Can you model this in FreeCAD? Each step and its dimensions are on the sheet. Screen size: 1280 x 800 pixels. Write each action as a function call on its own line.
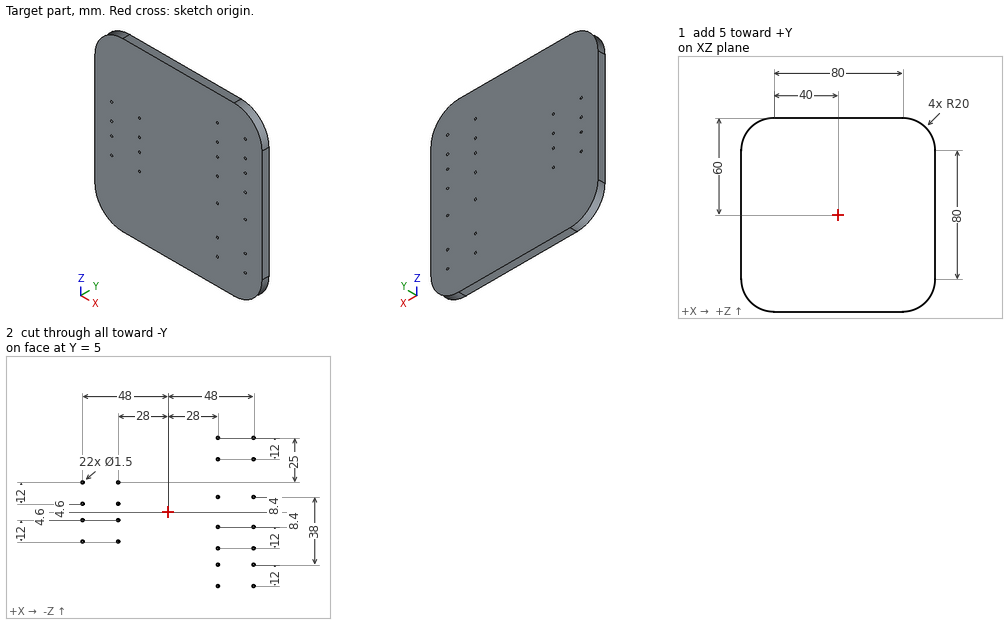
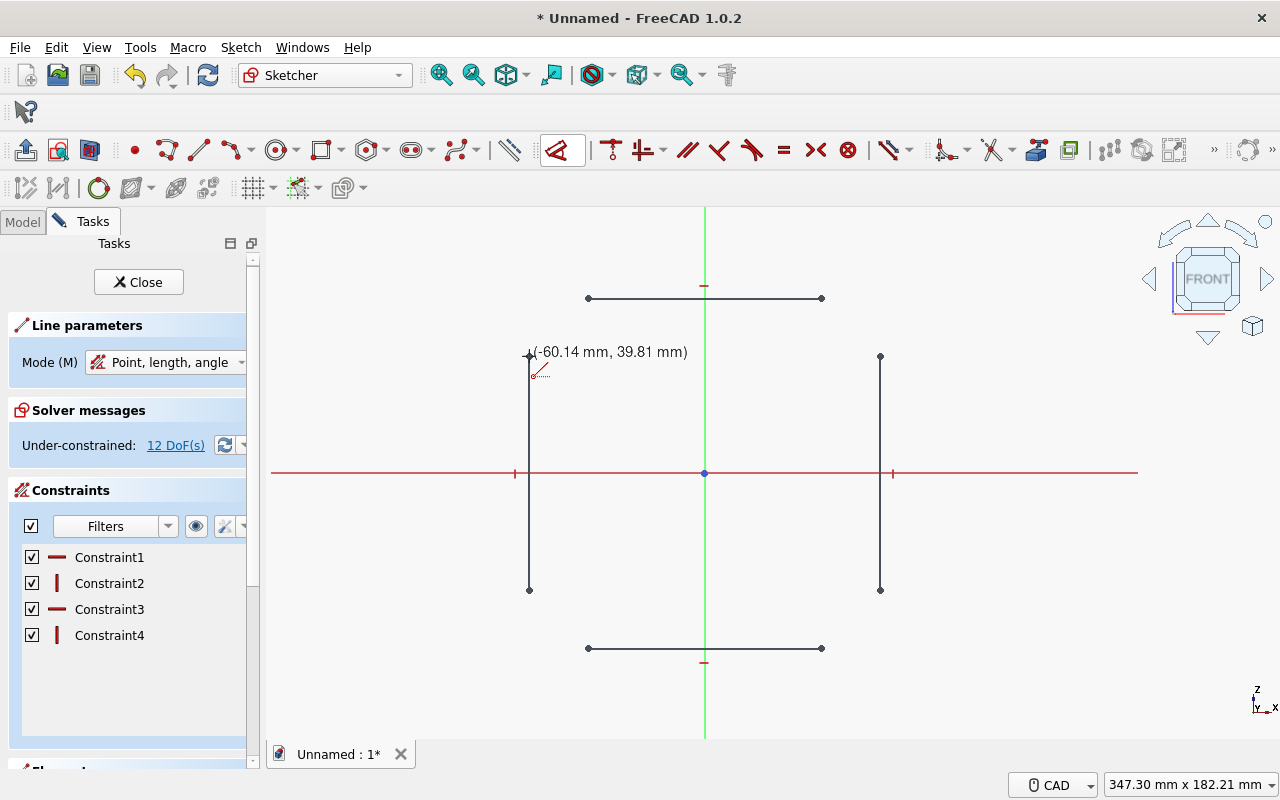
click(232, 150)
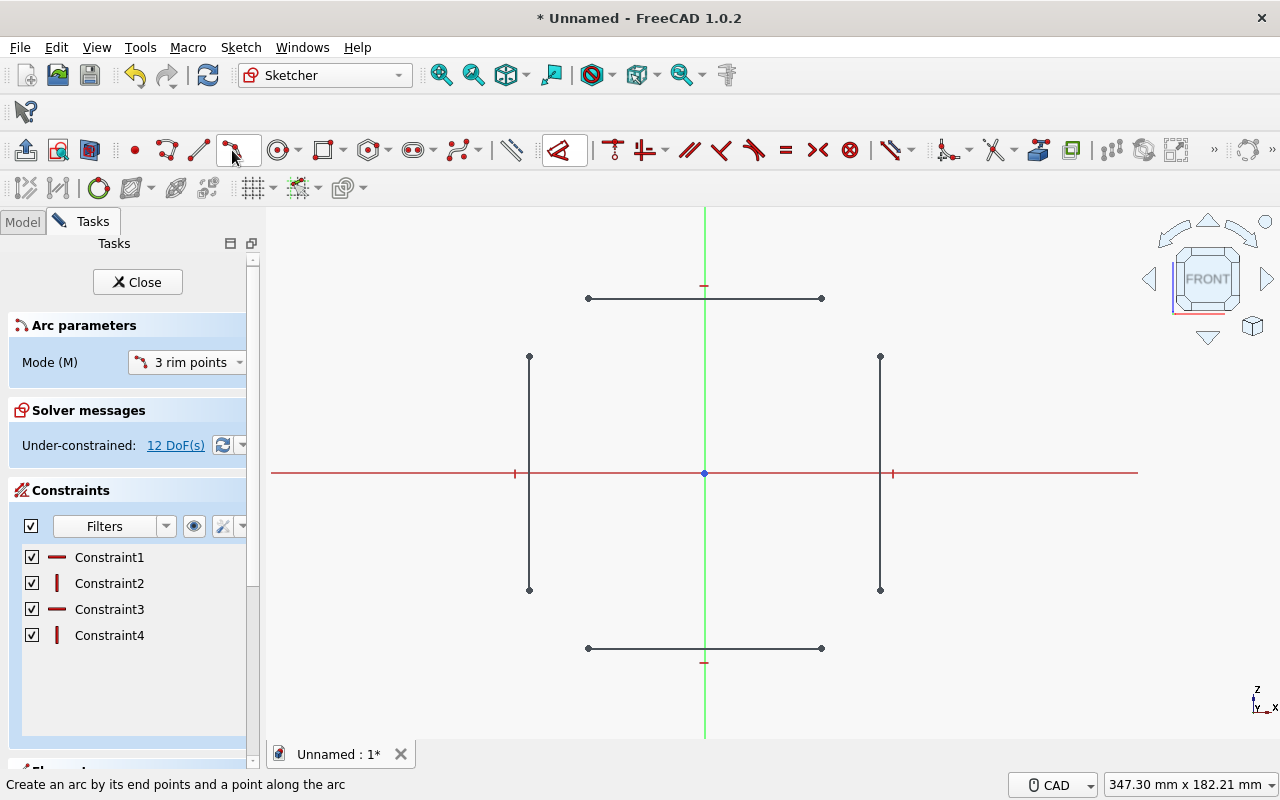
click(821, 299)
click(880, 357)
click(863, 315)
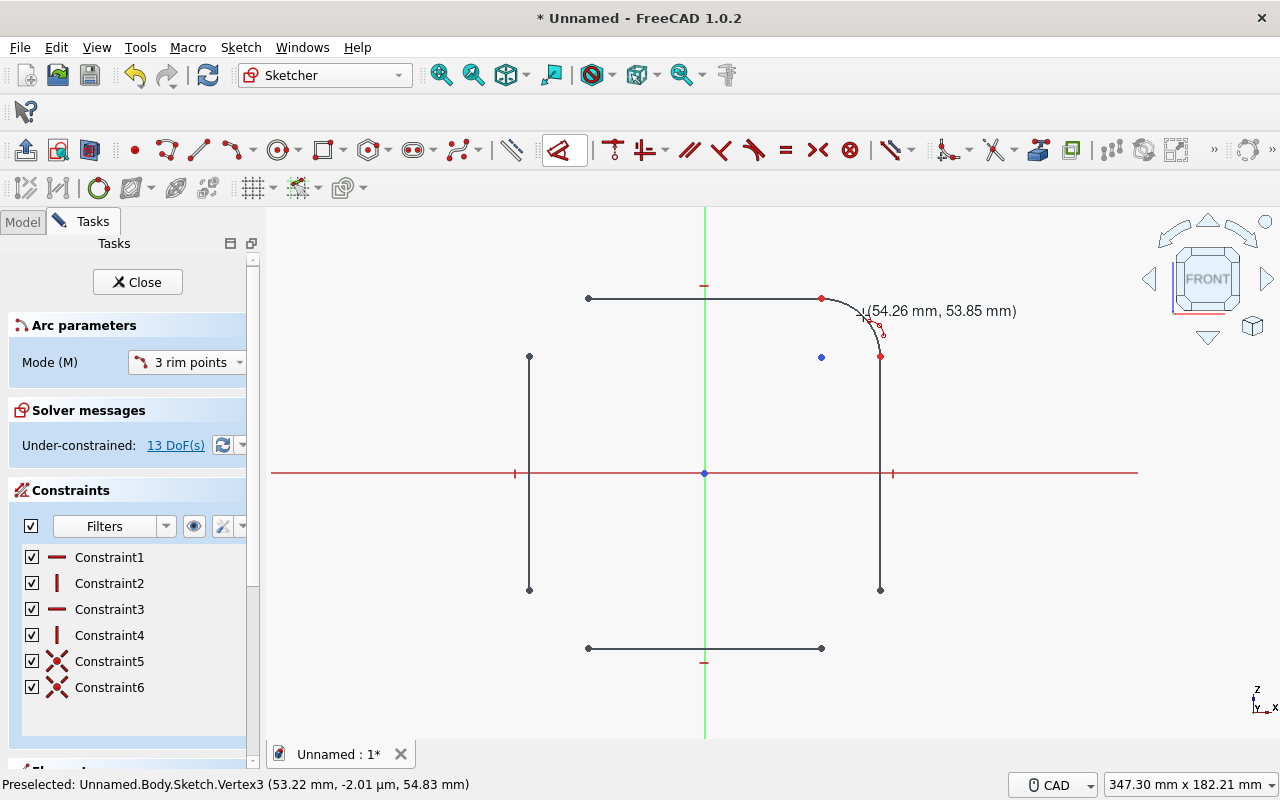
click(880, 591)
click(821, 649)
click(863, 631)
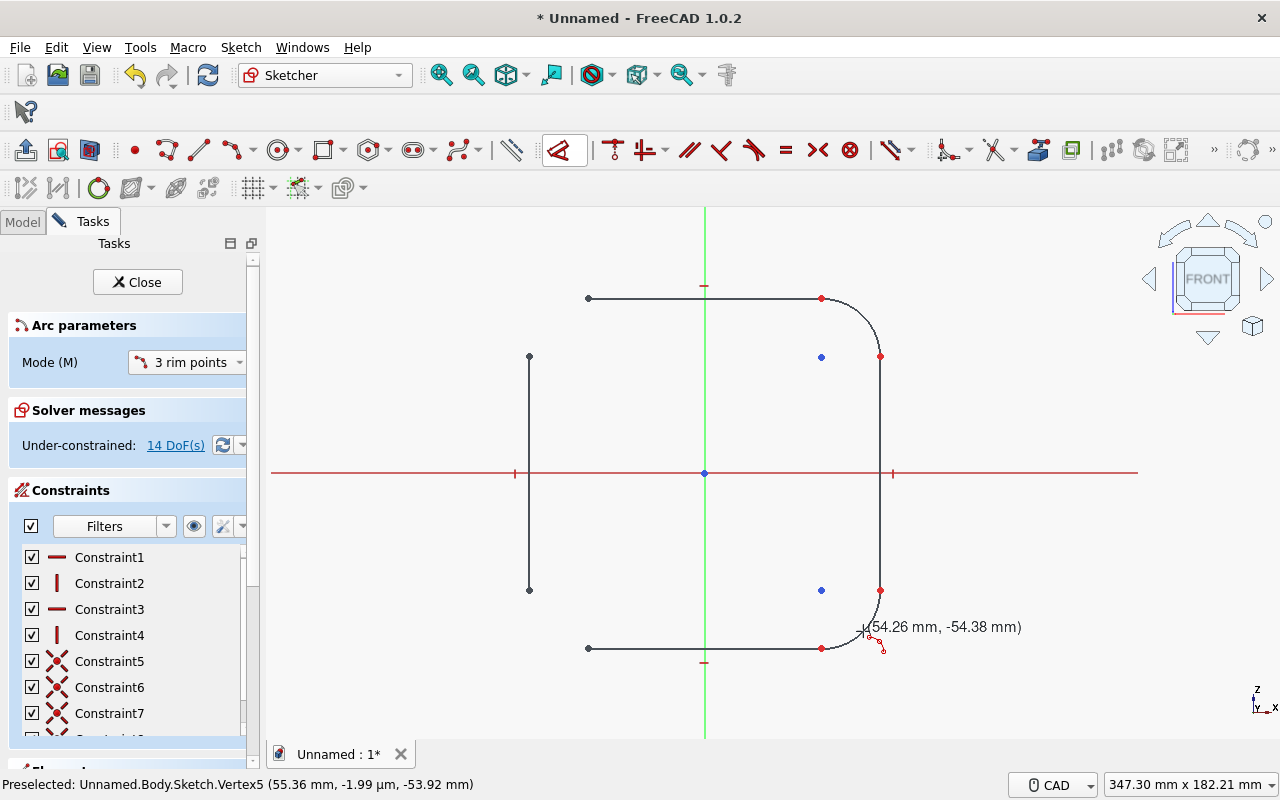
click(588, 649)
click(529, 591)
click(546, 631)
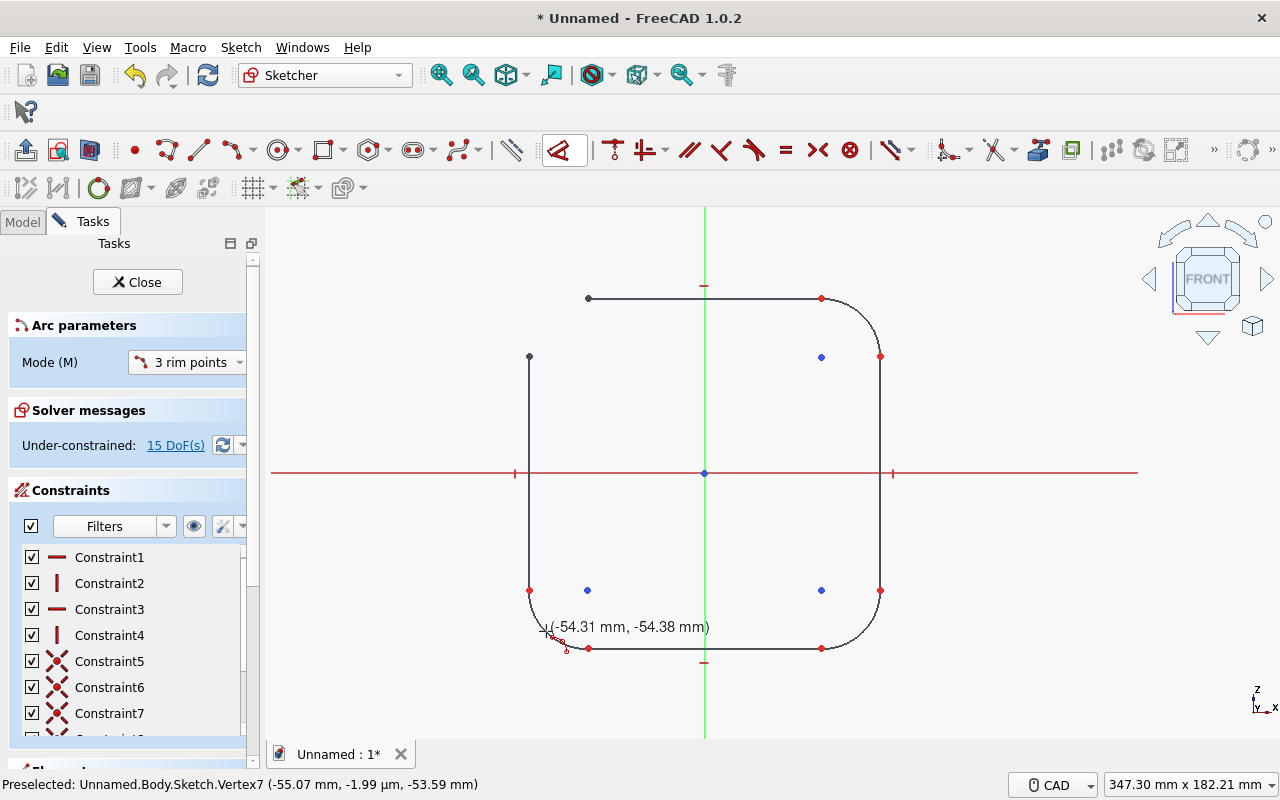
click(529, 357)
click(588, 299)
click(546, 315)
key(Escape)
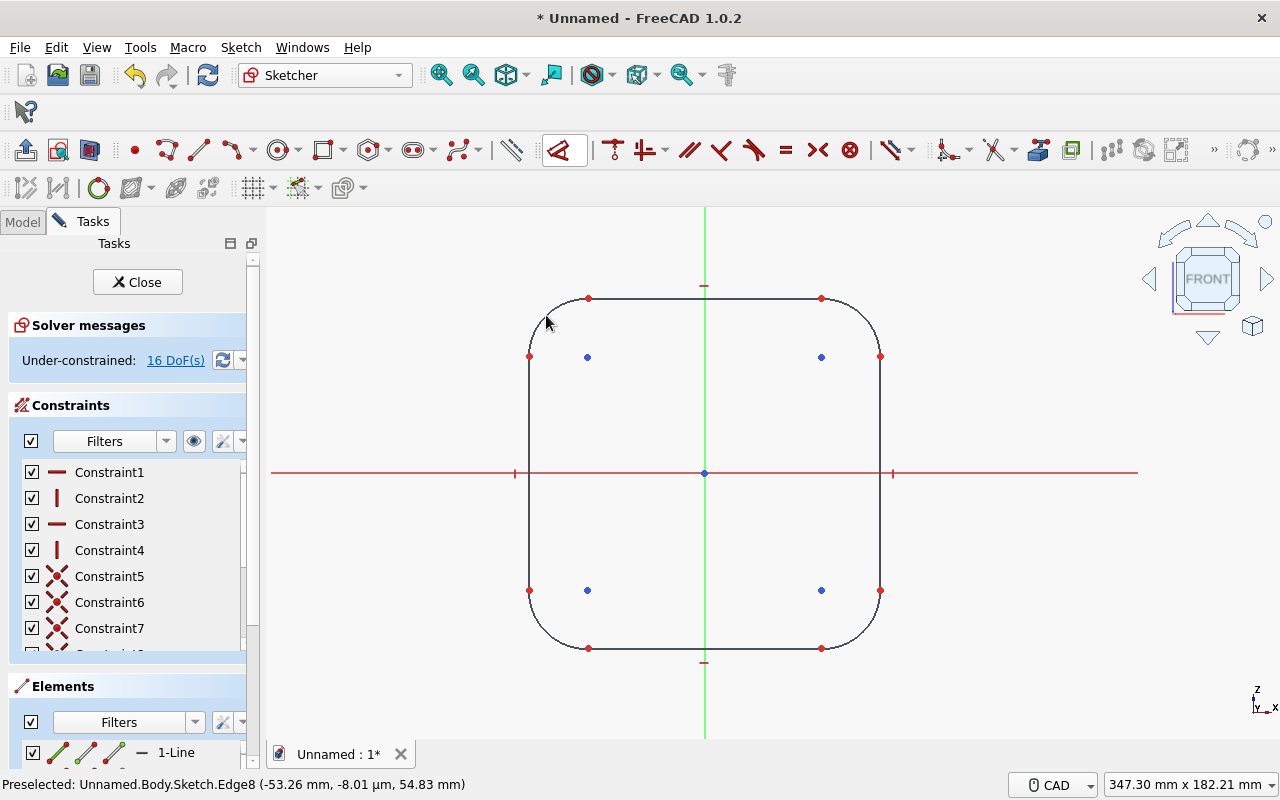
click(658, 299)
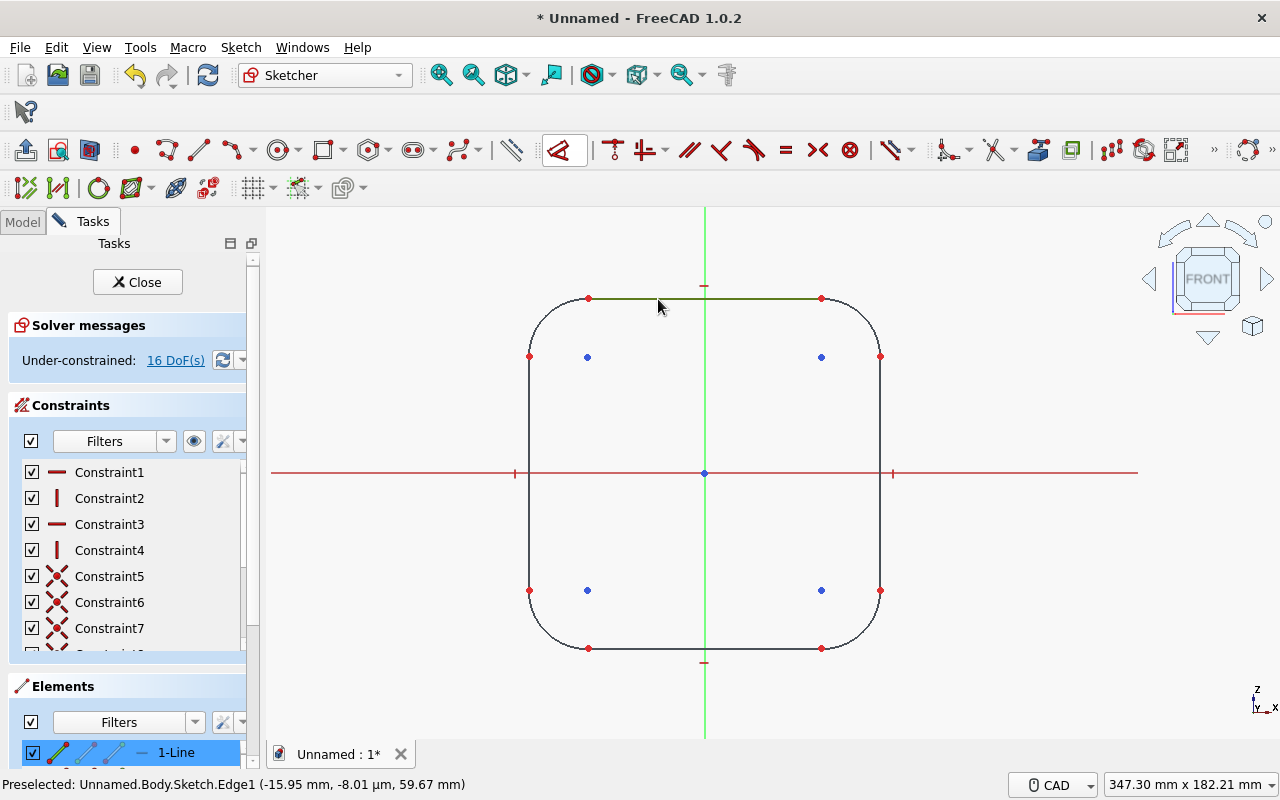
click(874, 330)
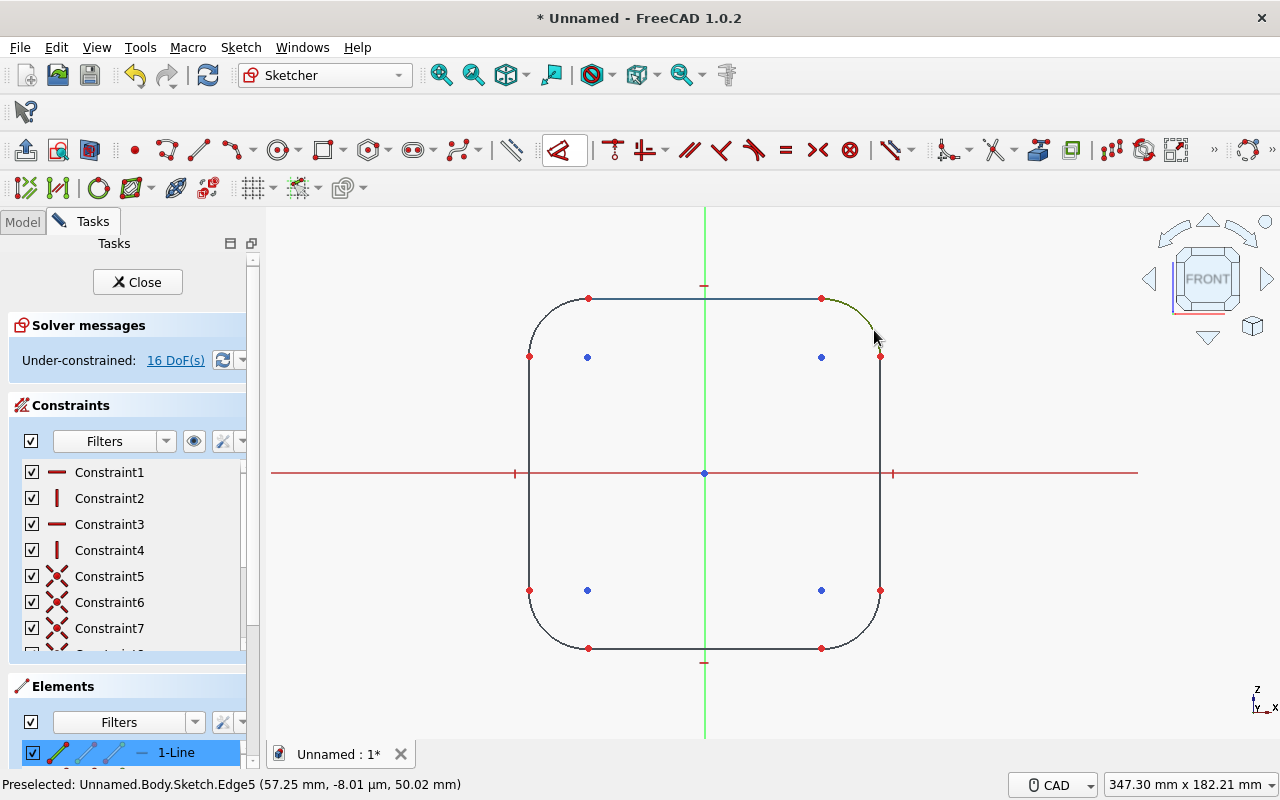
click(754, 150)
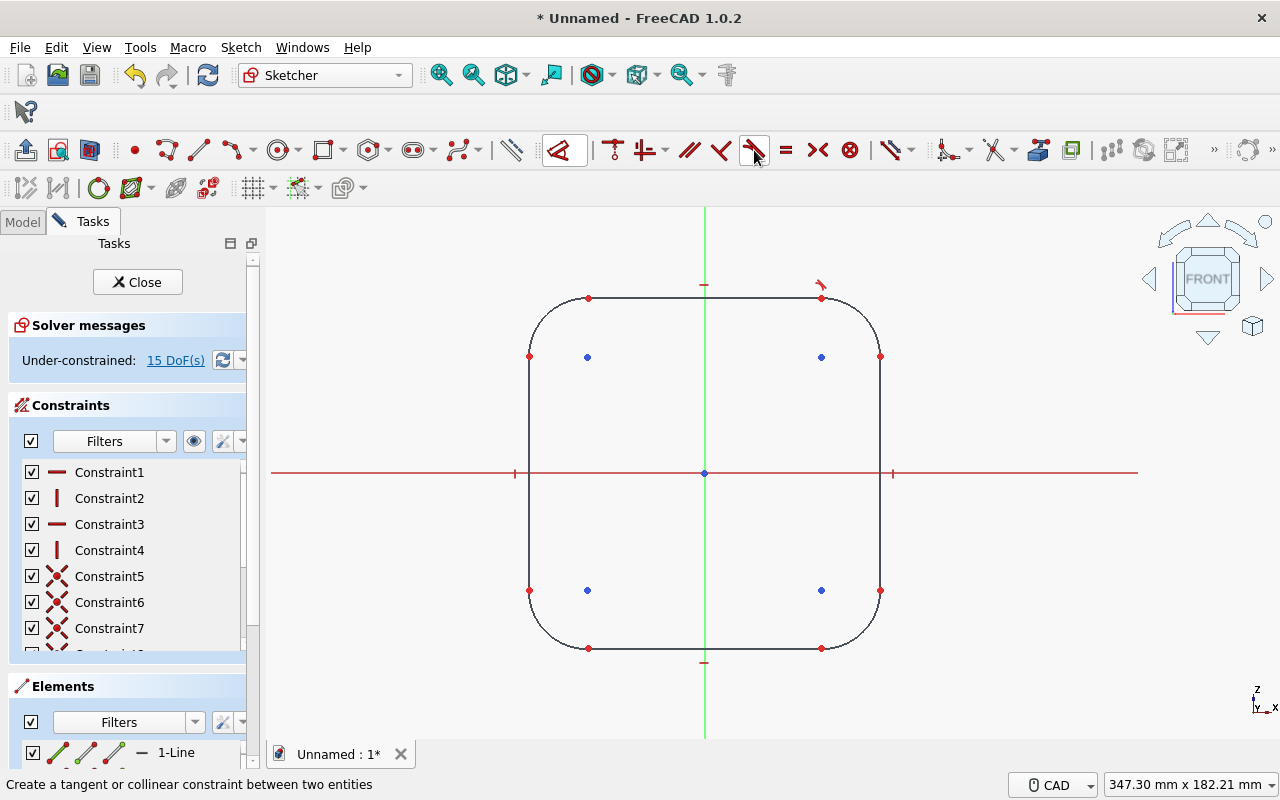
click(658, 298)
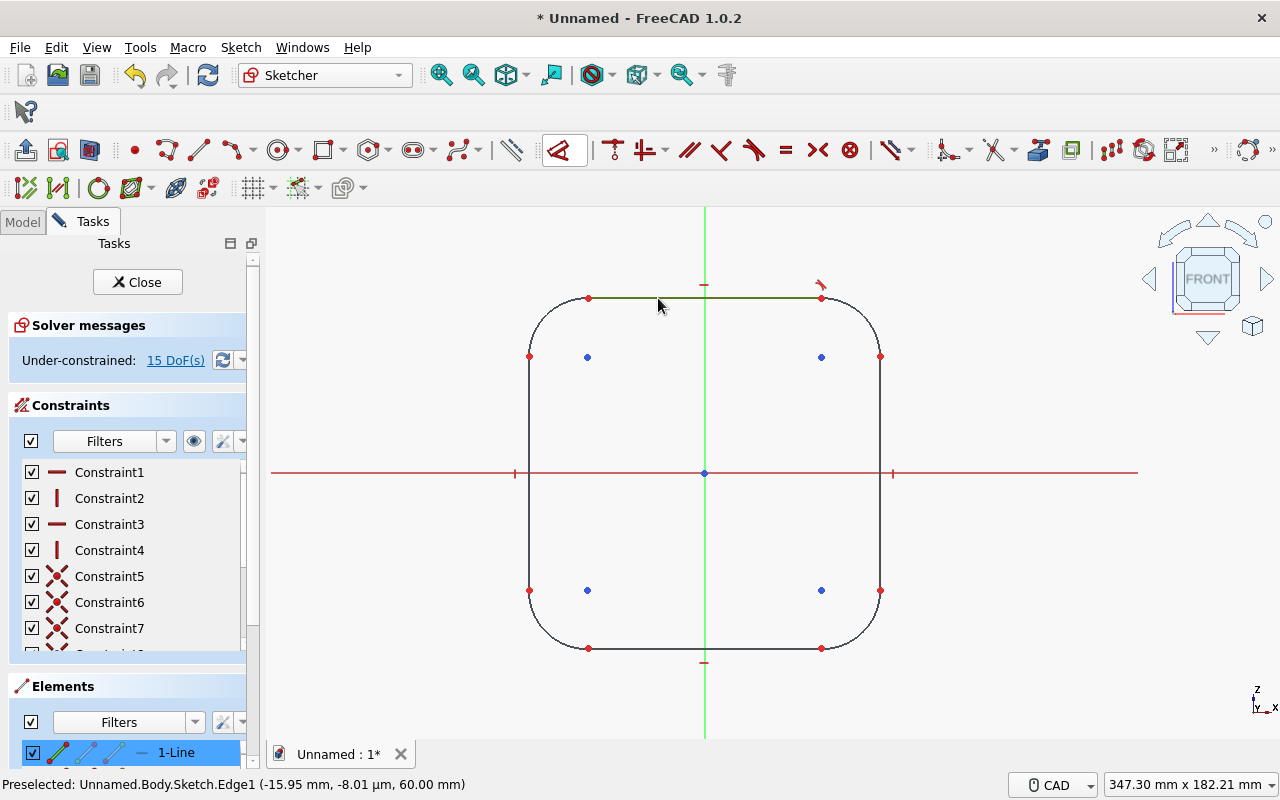
click(561, 304)